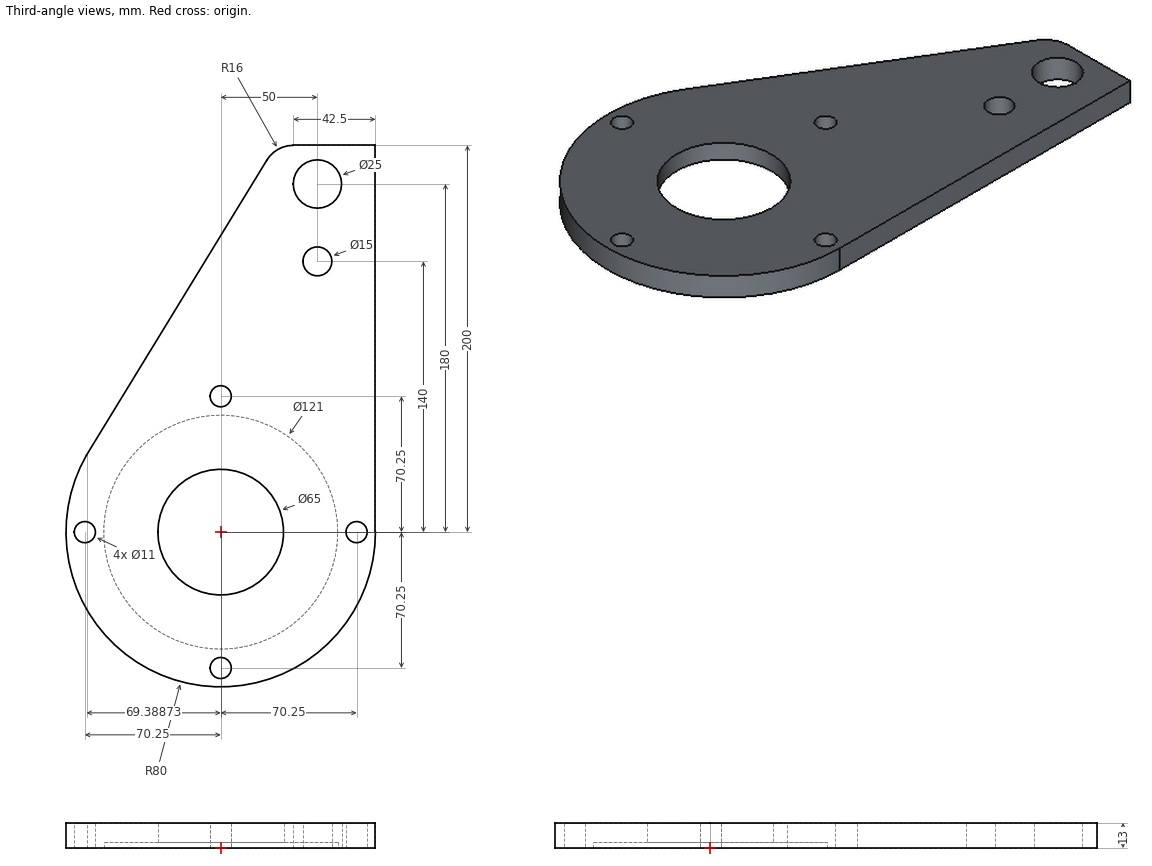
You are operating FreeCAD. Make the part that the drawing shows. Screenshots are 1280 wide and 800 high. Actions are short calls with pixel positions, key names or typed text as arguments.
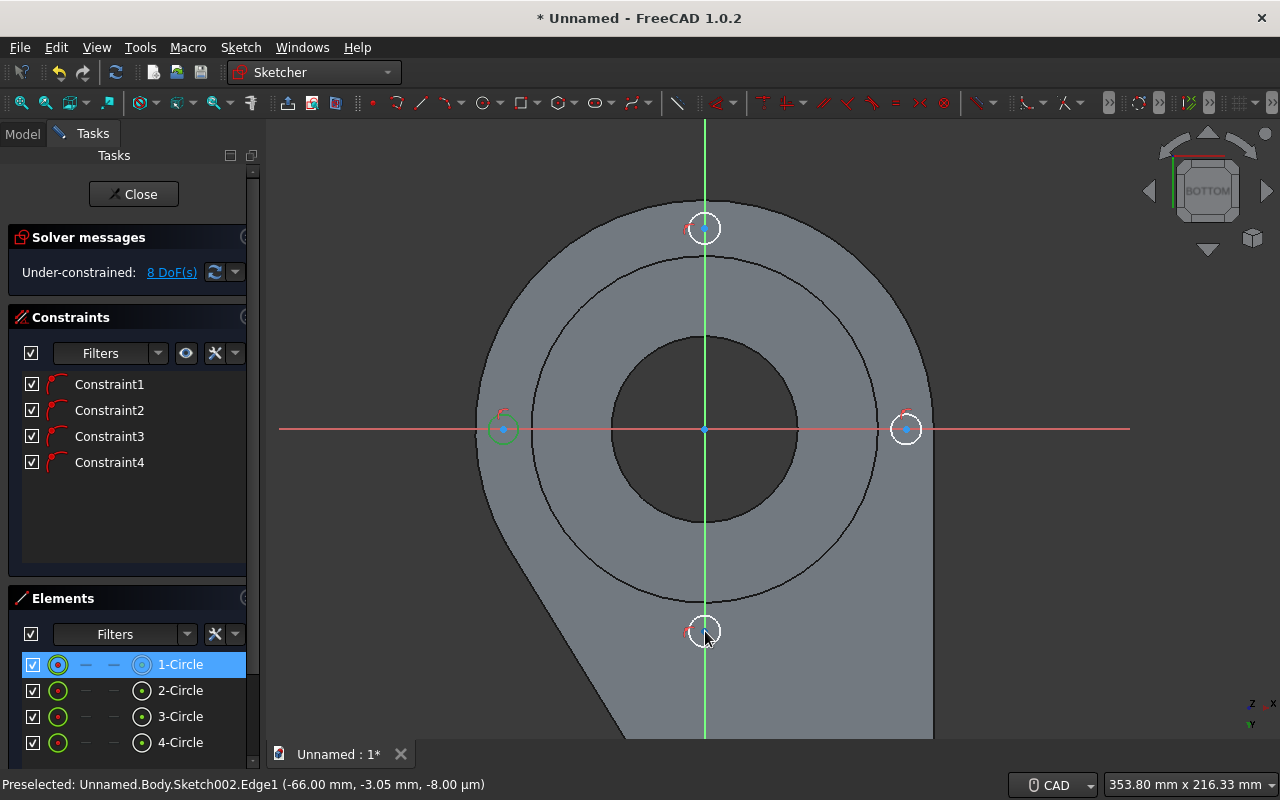
scroll(716, 217, up, 2)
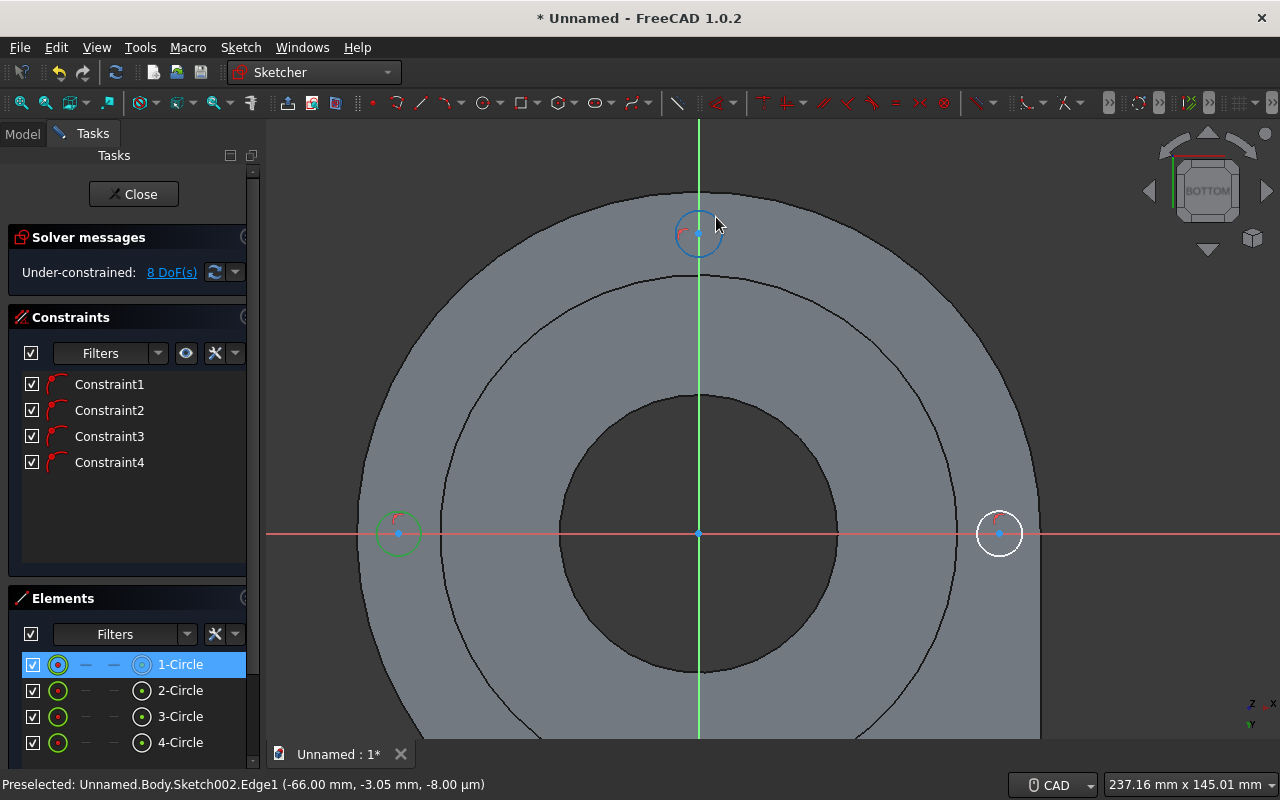
click(715, 217)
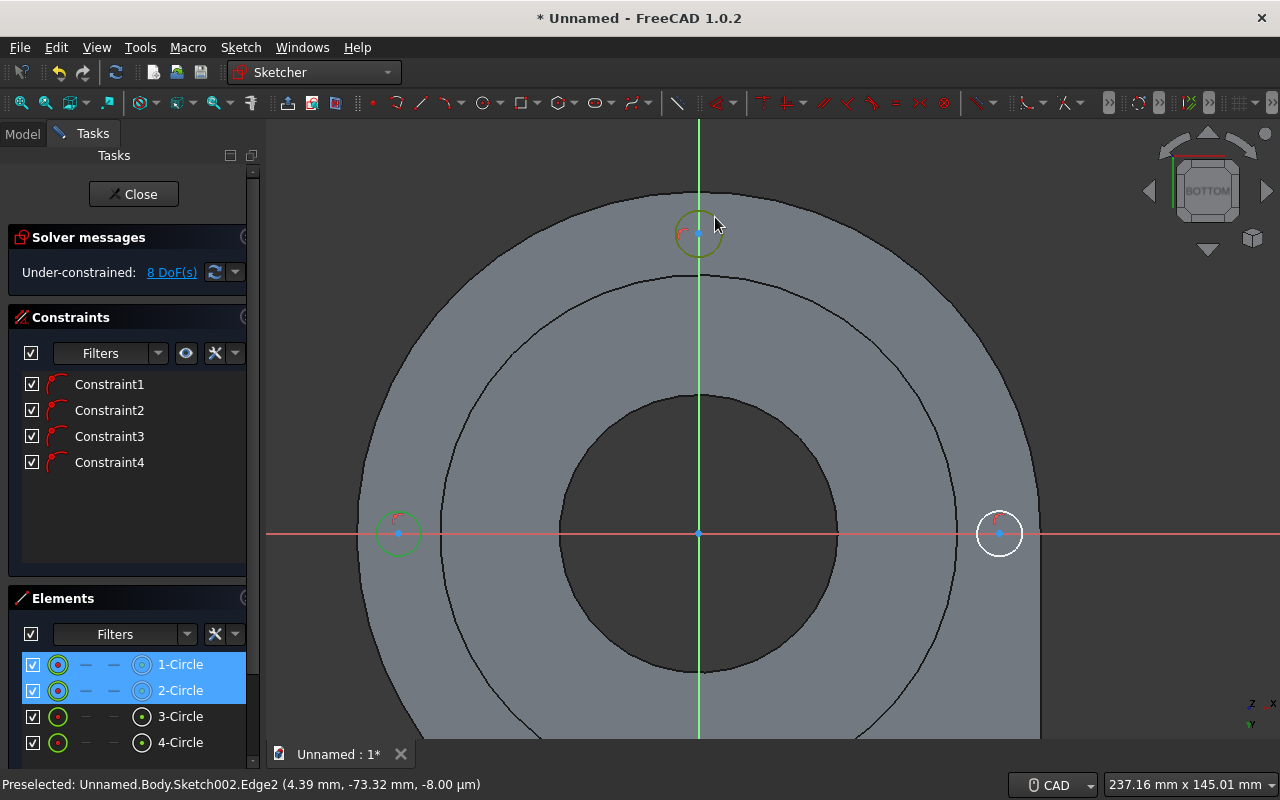
click(1015, 518)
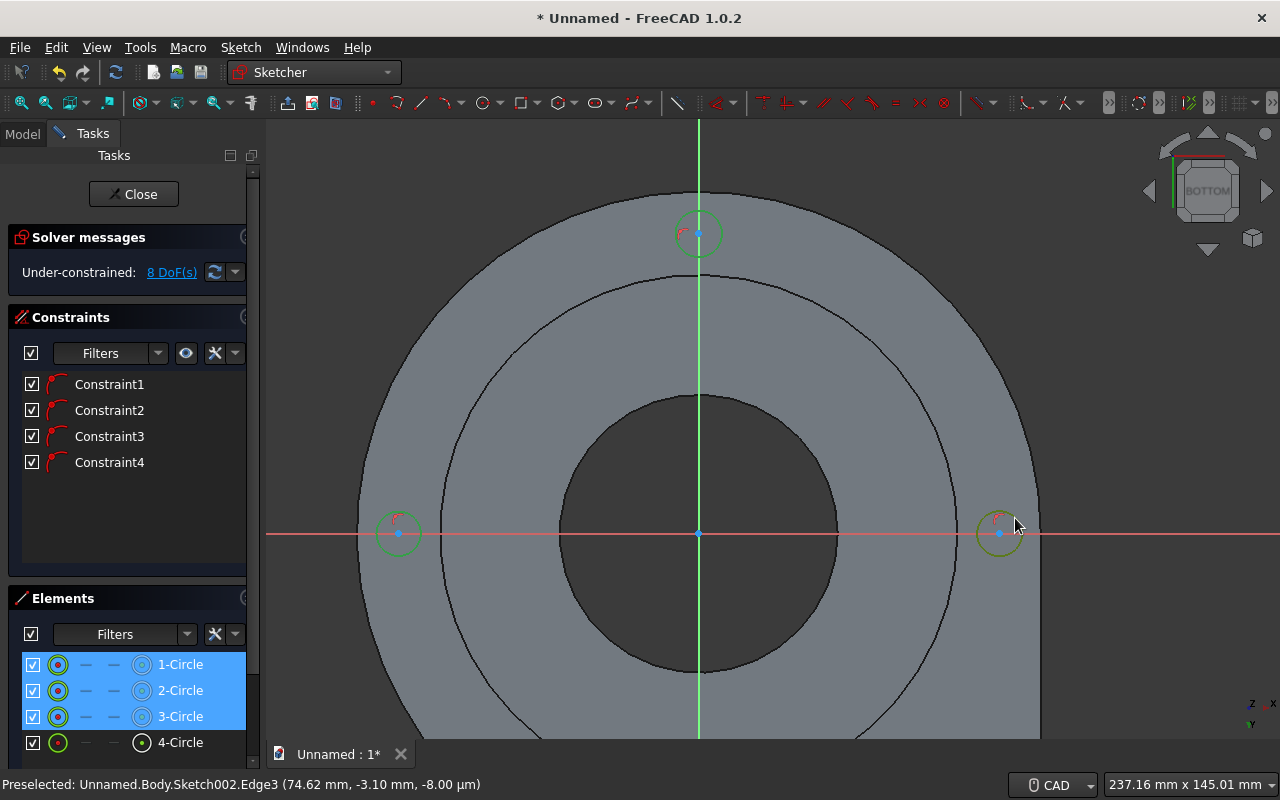
scroll(716, 216, down, 2)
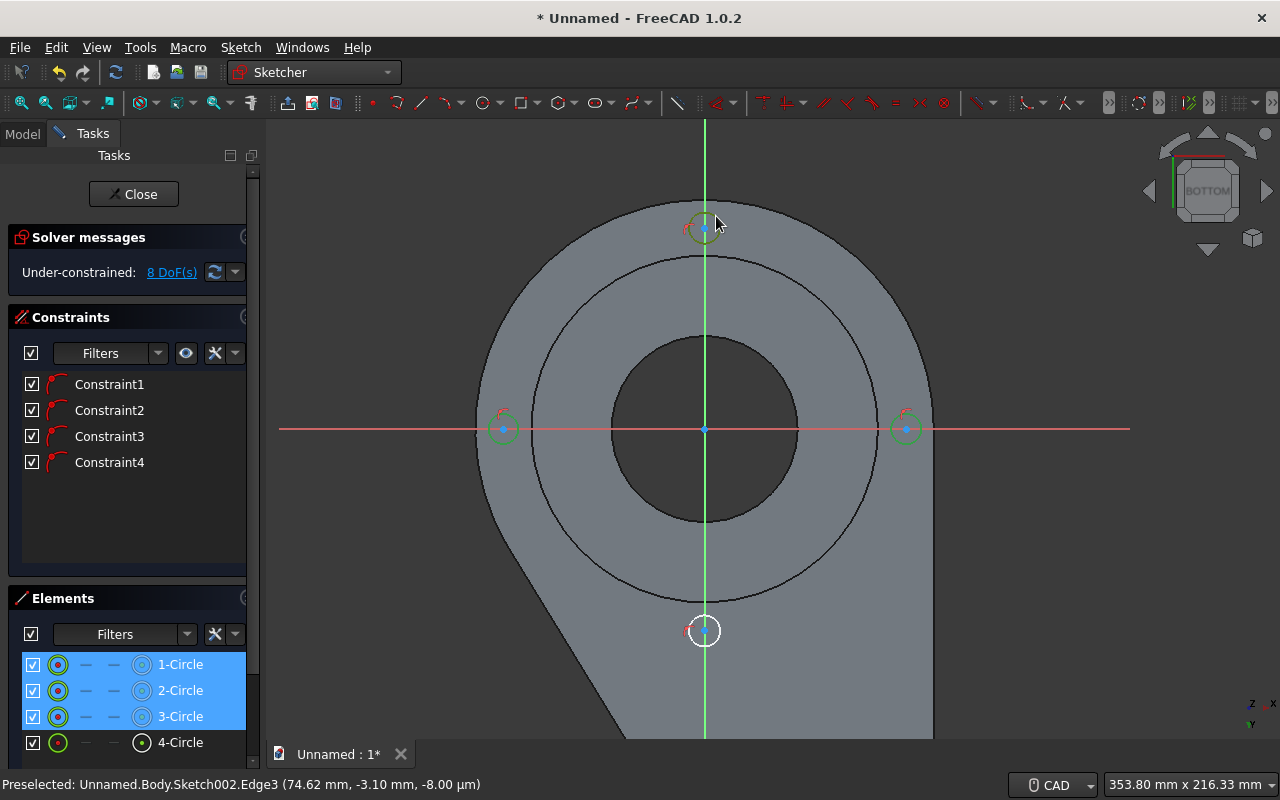
scroll(716, 620, up, 2)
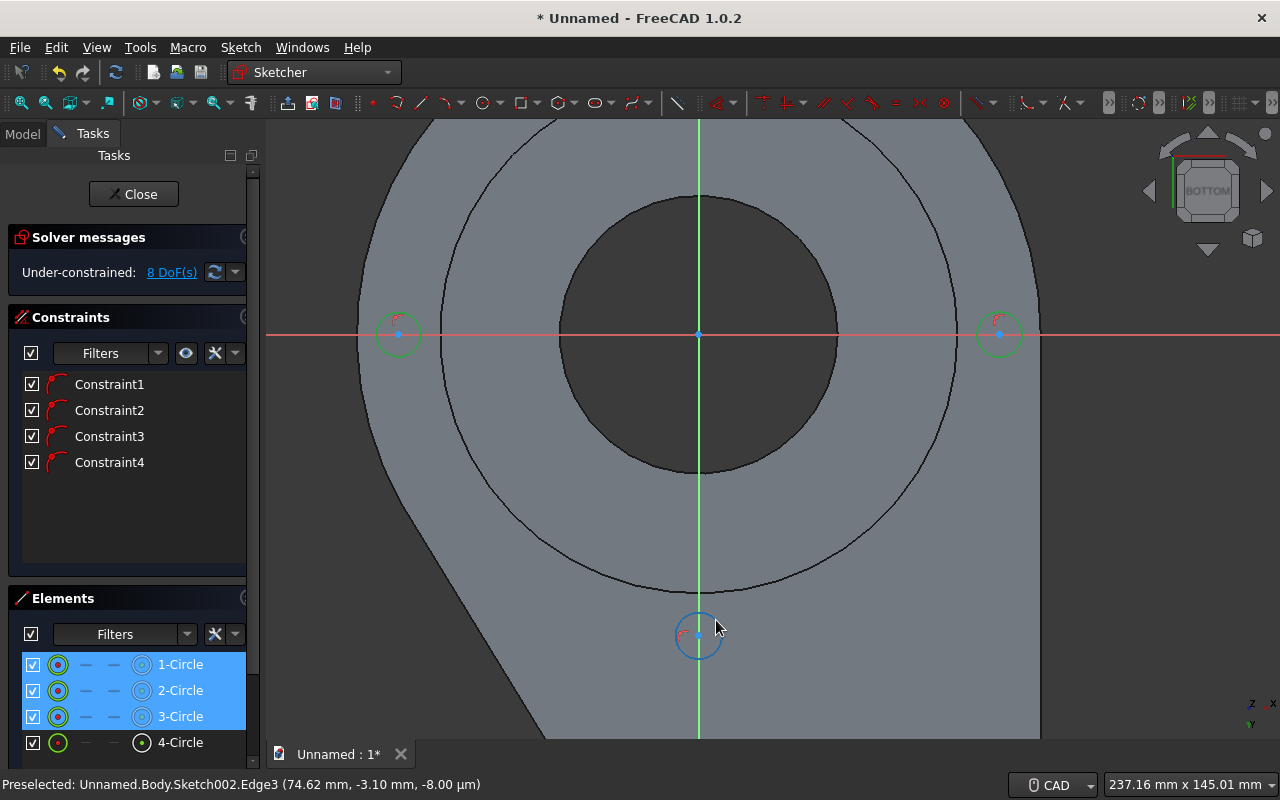
click(715, 619)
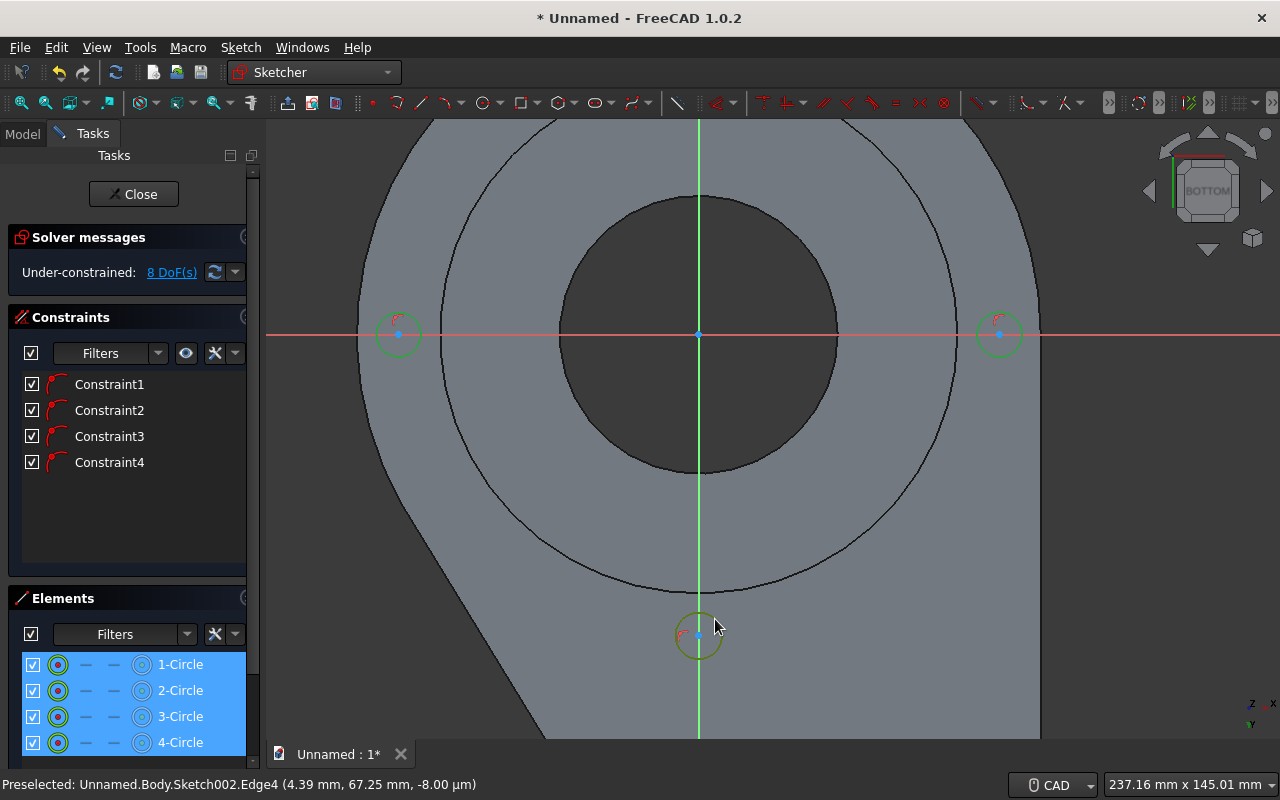
click(896, 104)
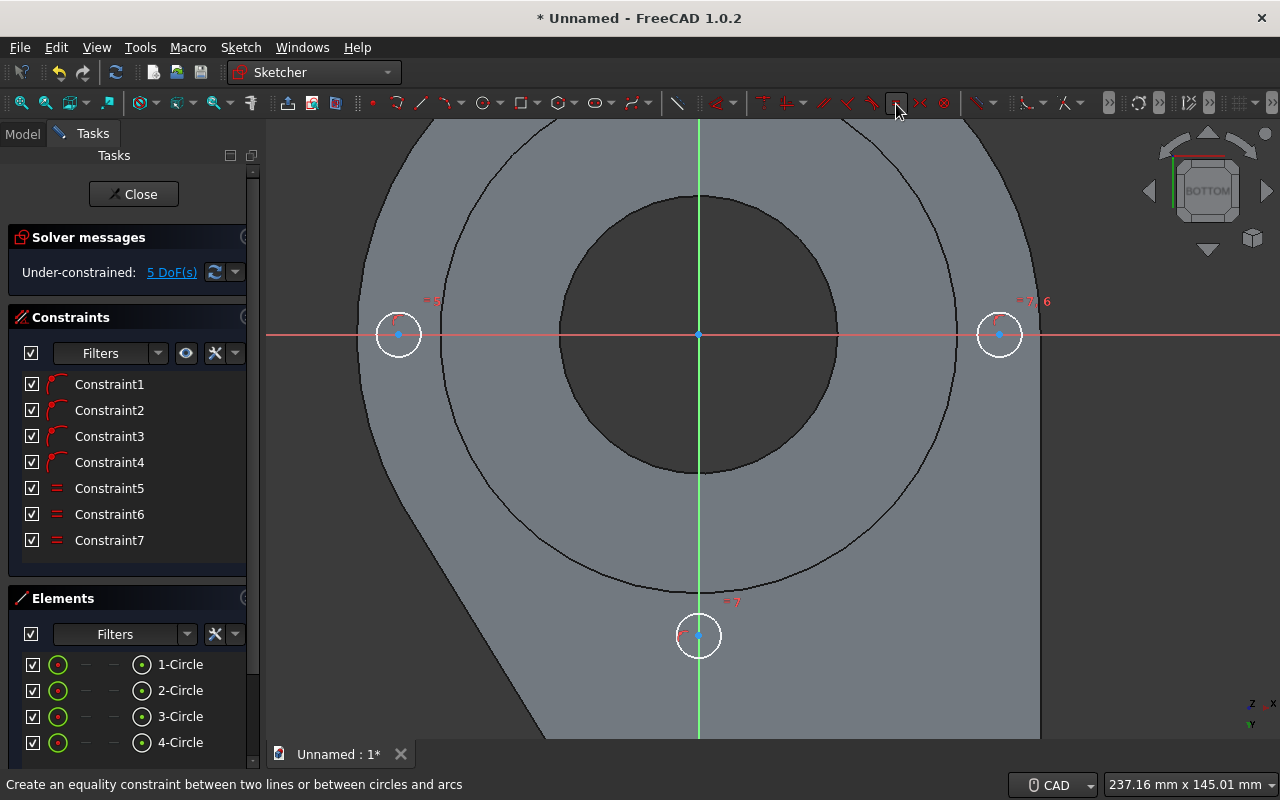
click(716, 104)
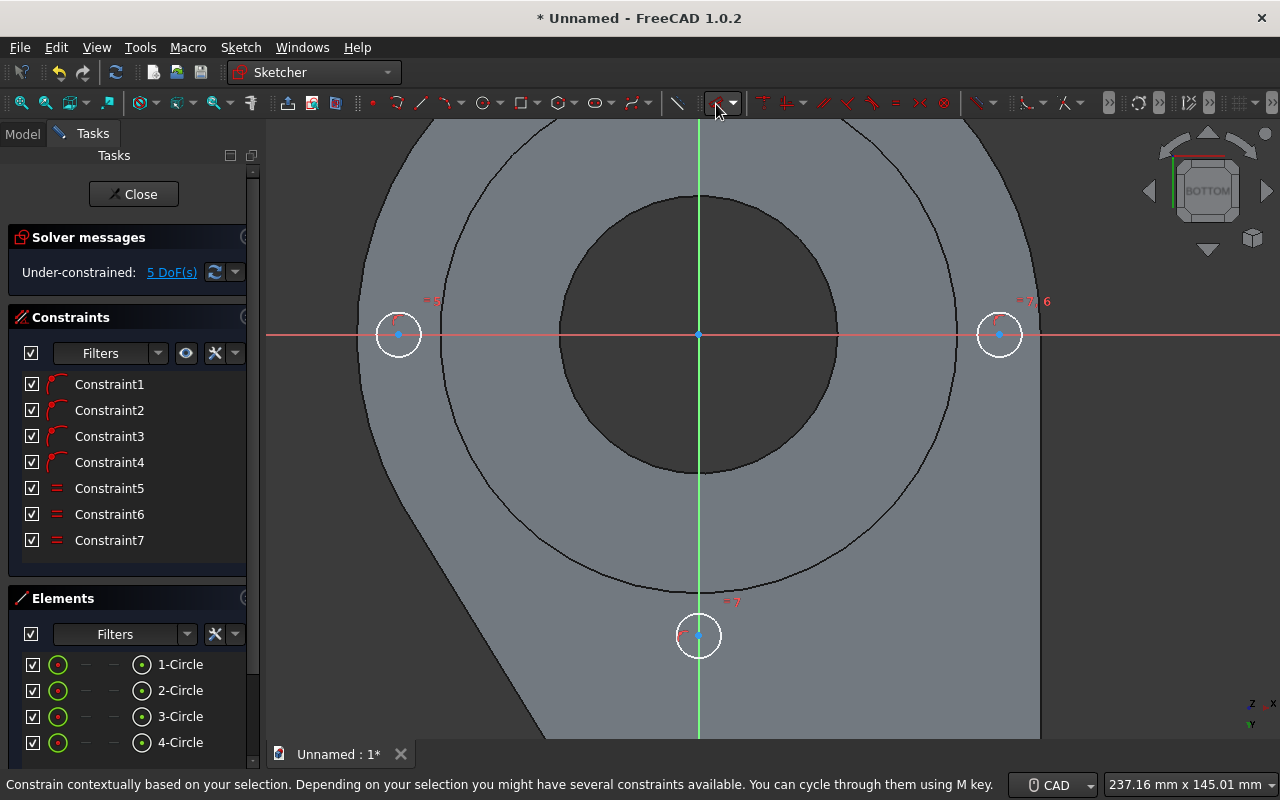
click(414, 319)
click(436, 296)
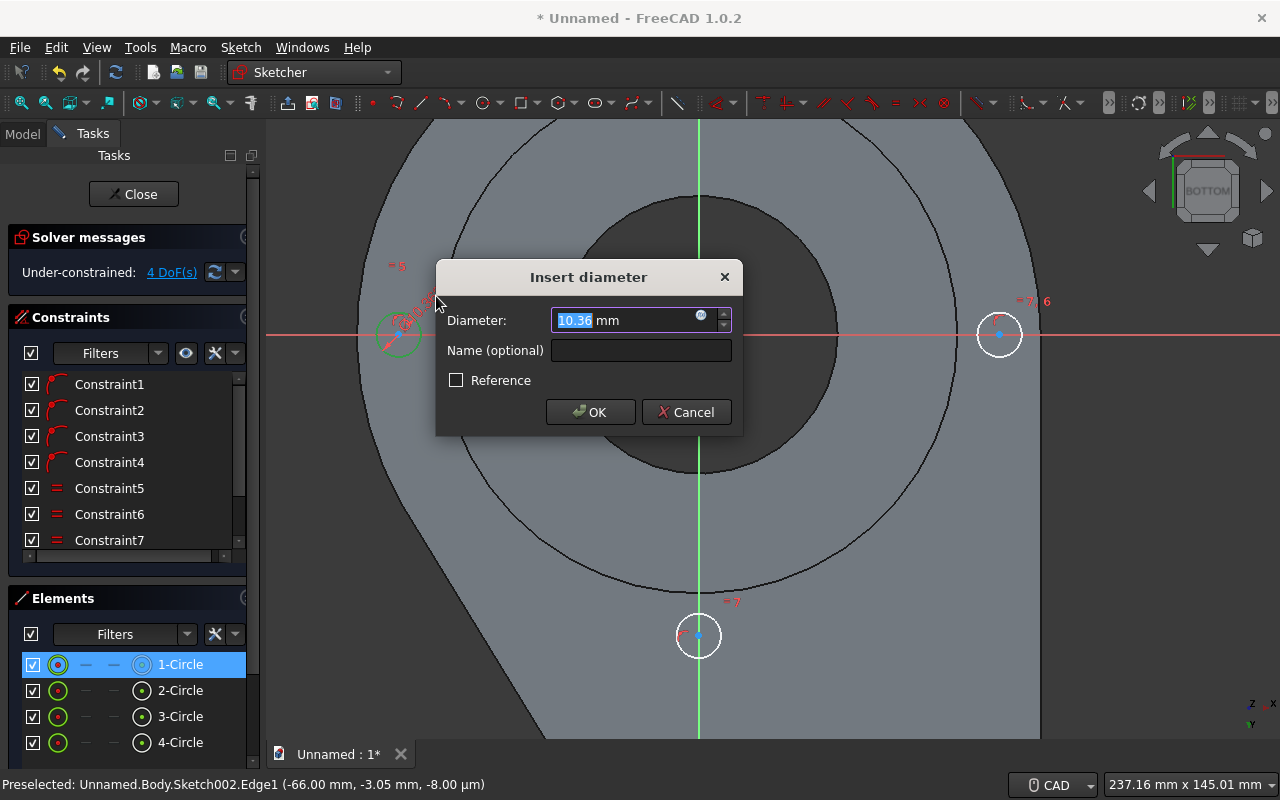
text(11)
key(Return)